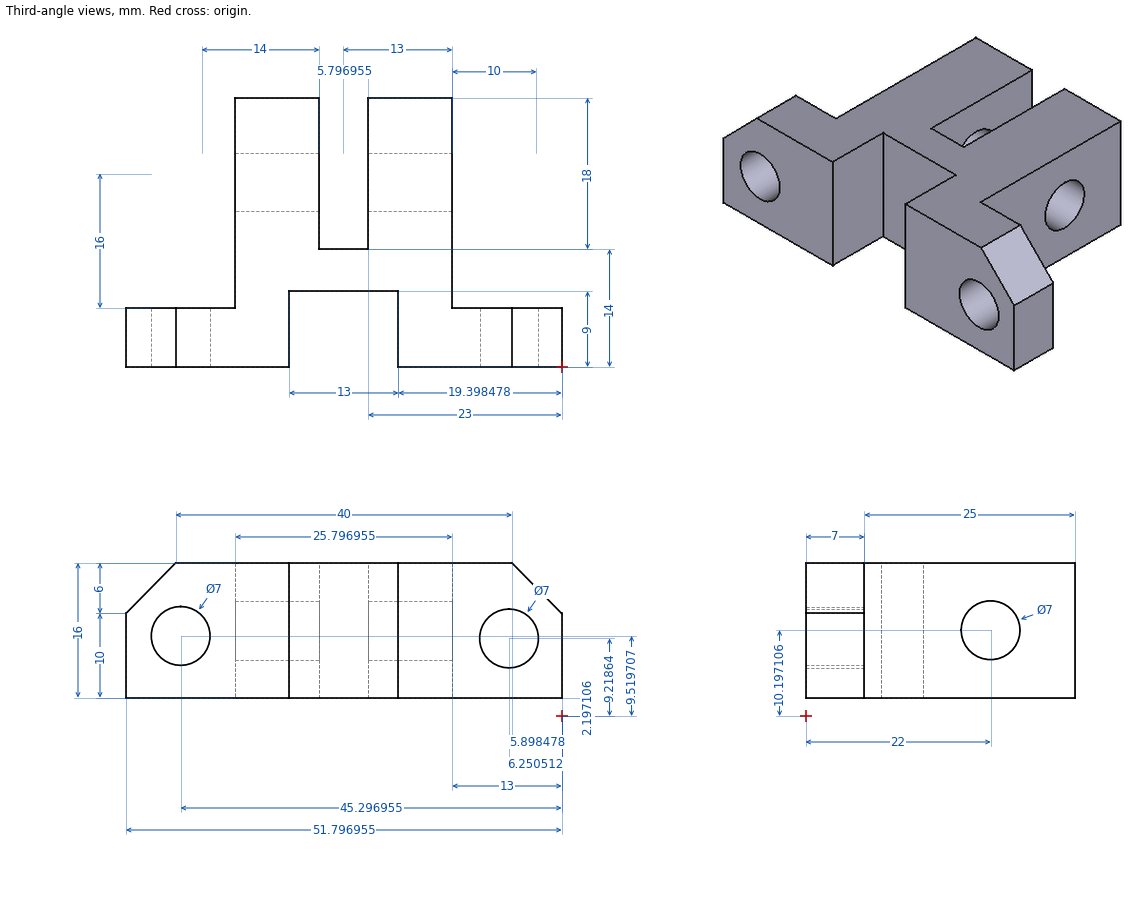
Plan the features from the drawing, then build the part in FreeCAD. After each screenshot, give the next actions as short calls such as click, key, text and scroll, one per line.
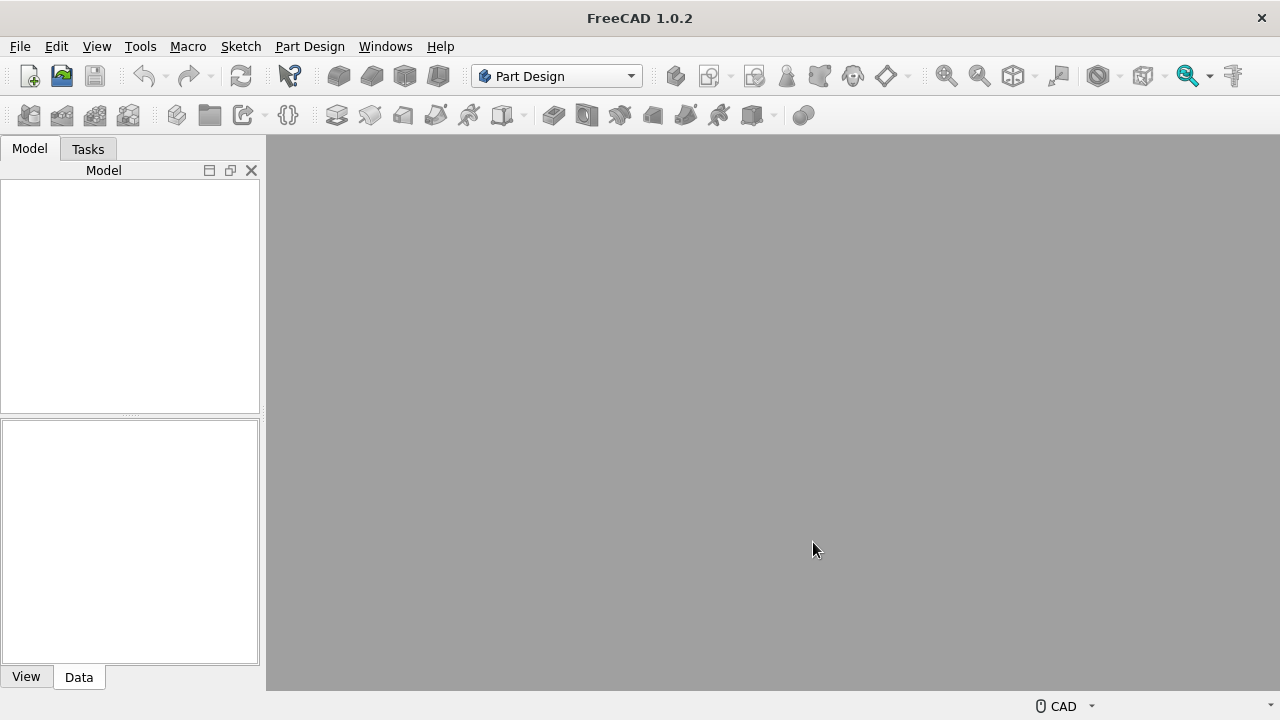
key(ctrl+n)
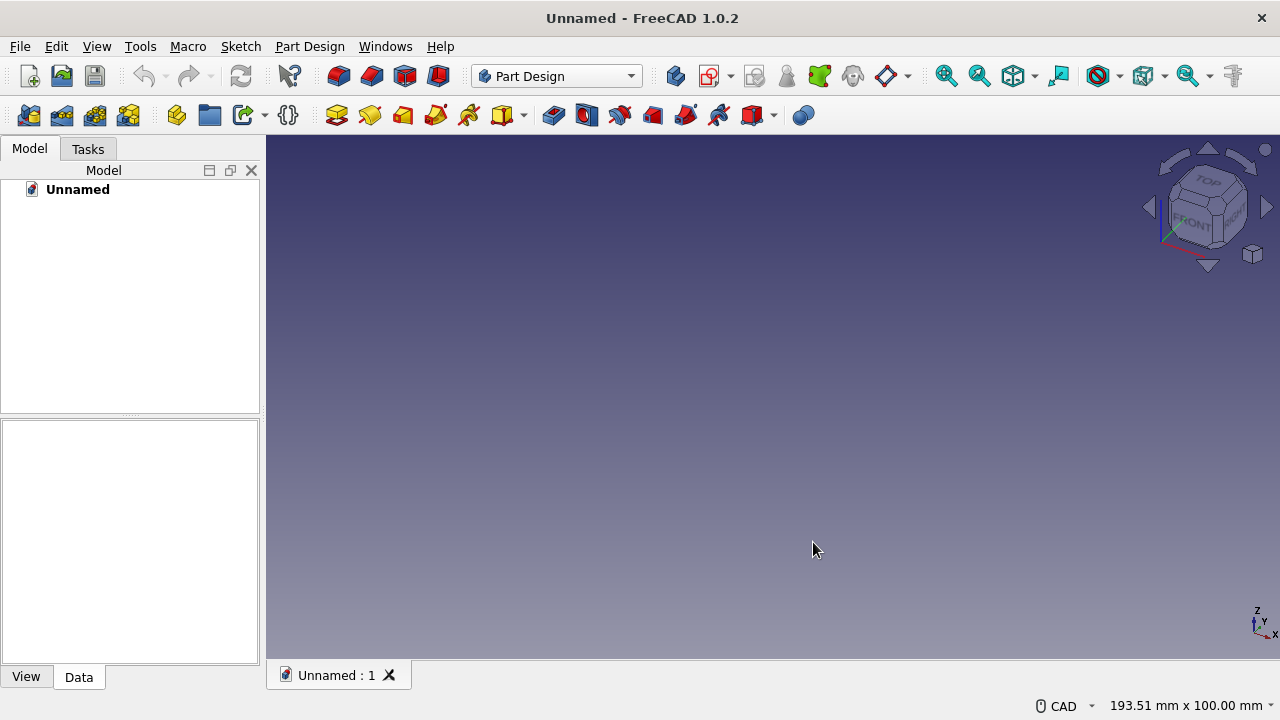
click(708, 76)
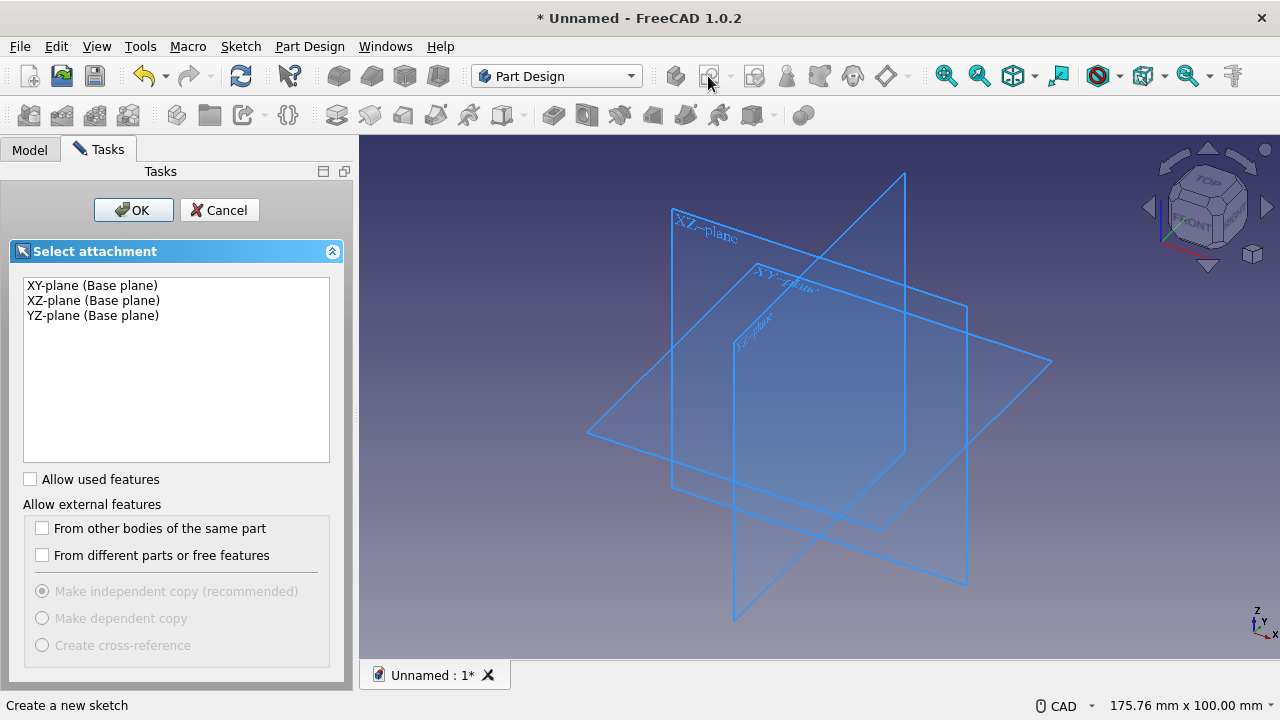
click(84, 300)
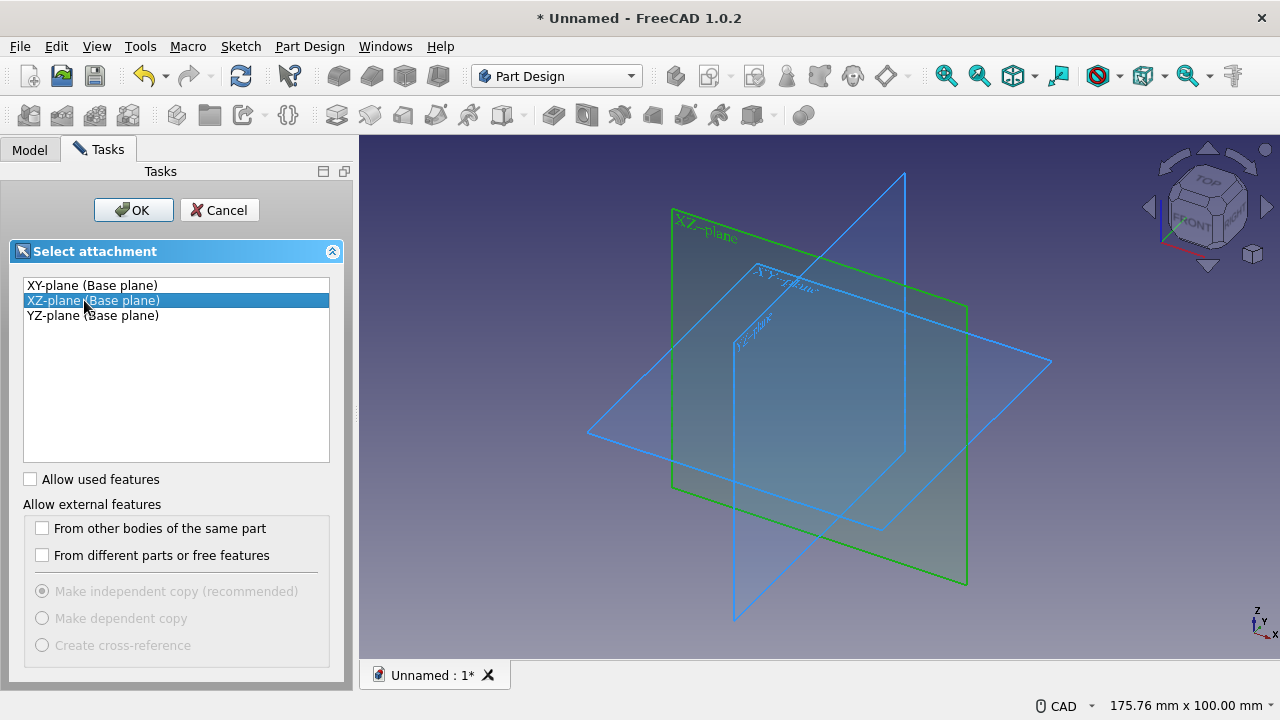
click(134, 210)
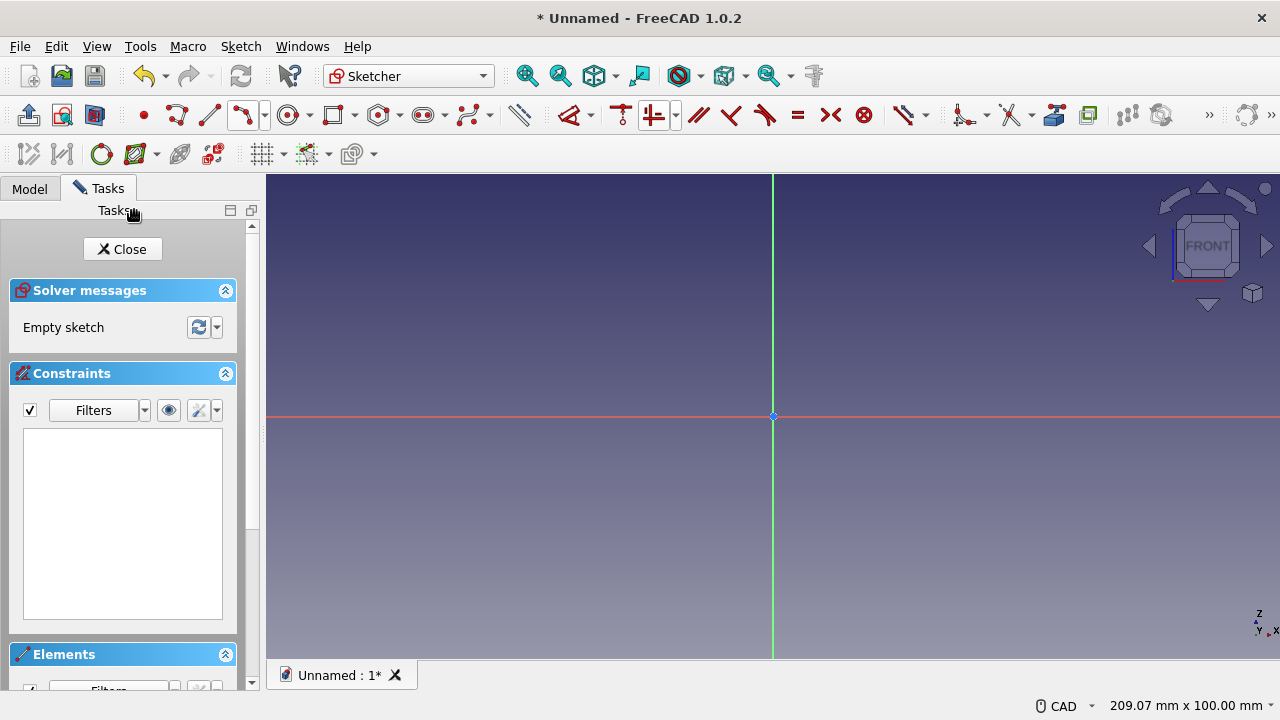
scroll(601, 336, up, 4)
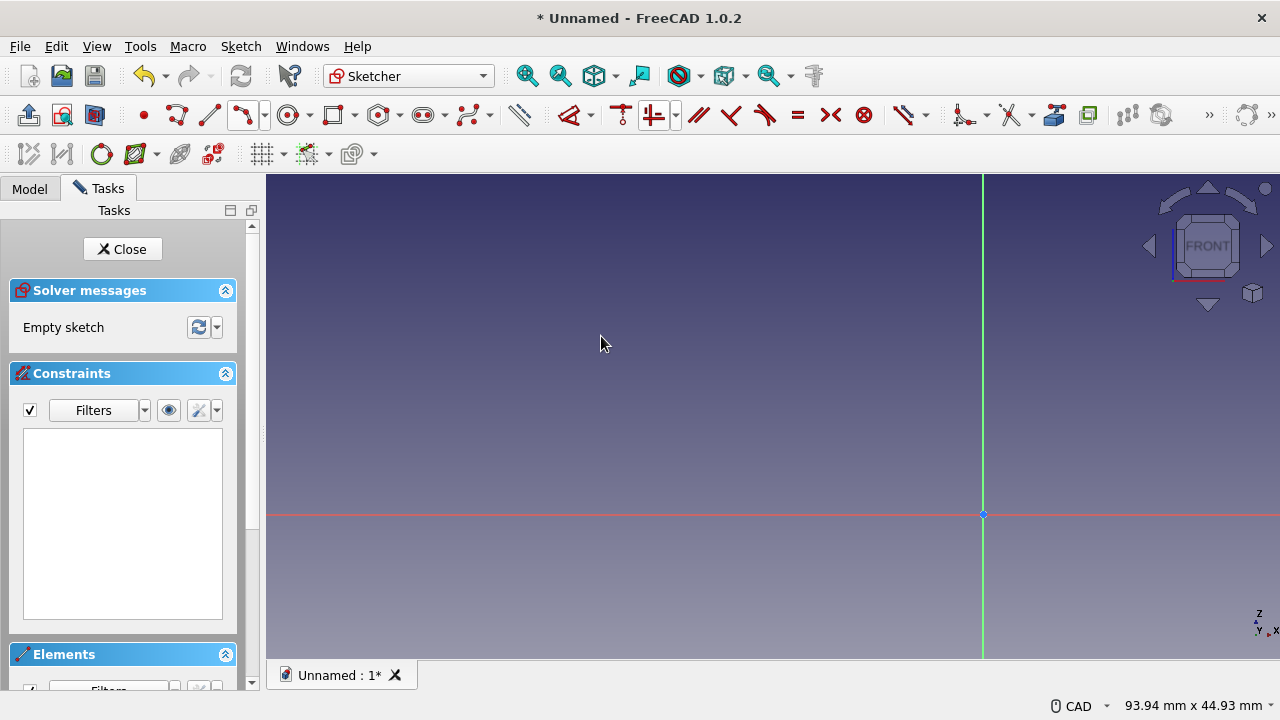
key(g)
key(m)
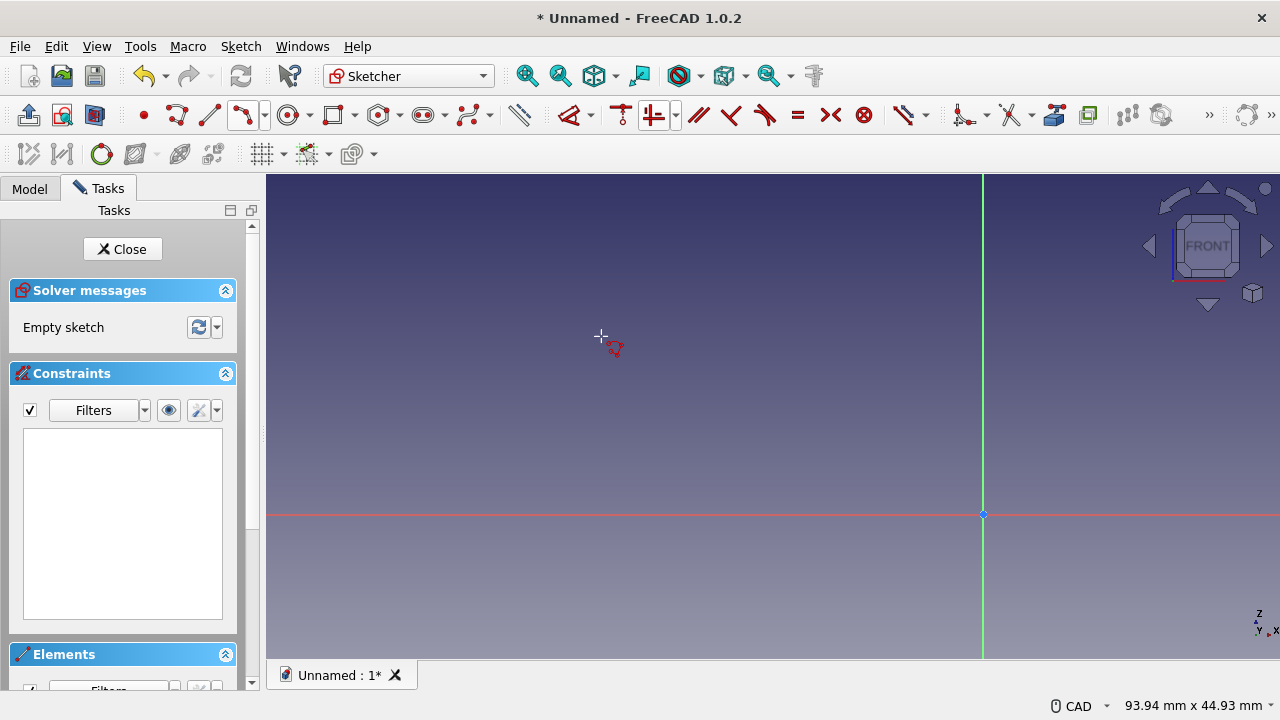
click(983, 491)
click(424, 491)
click(424, 383)
click(488, 318)
click(920, 318)
click(974, 383)
click(983, 492)
key(Escape)
key(Escape)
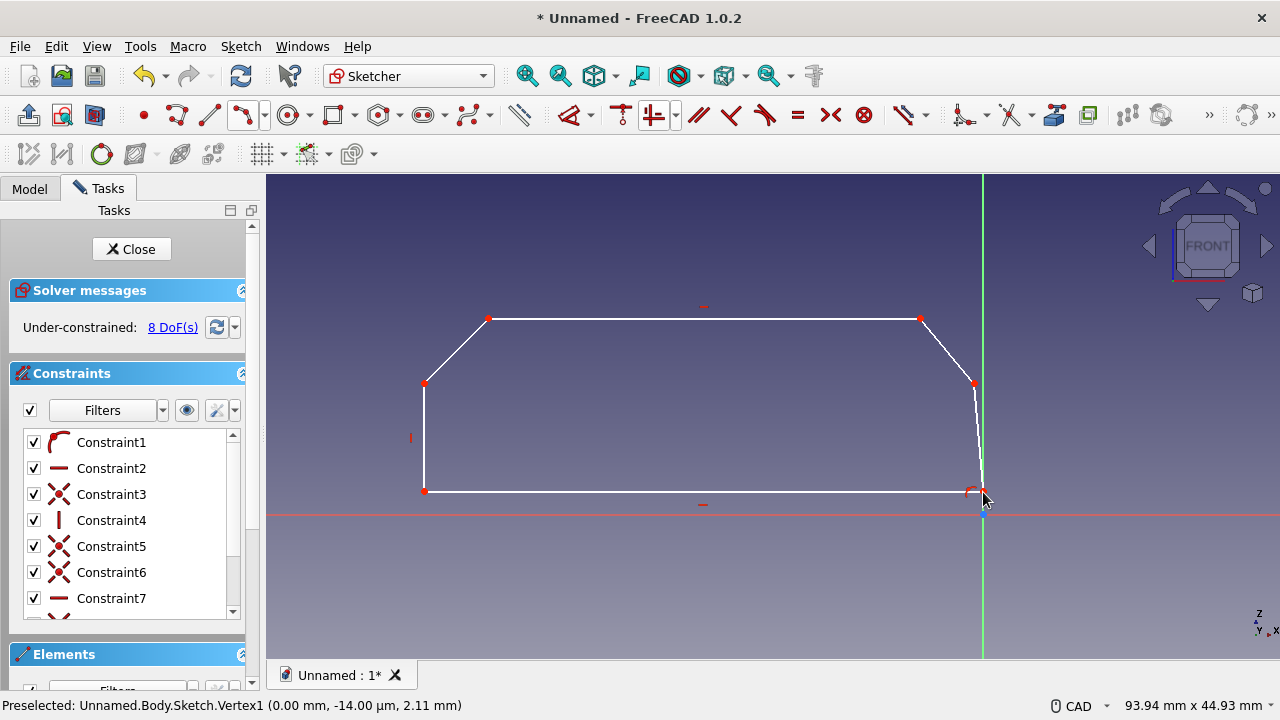
click(981, 460)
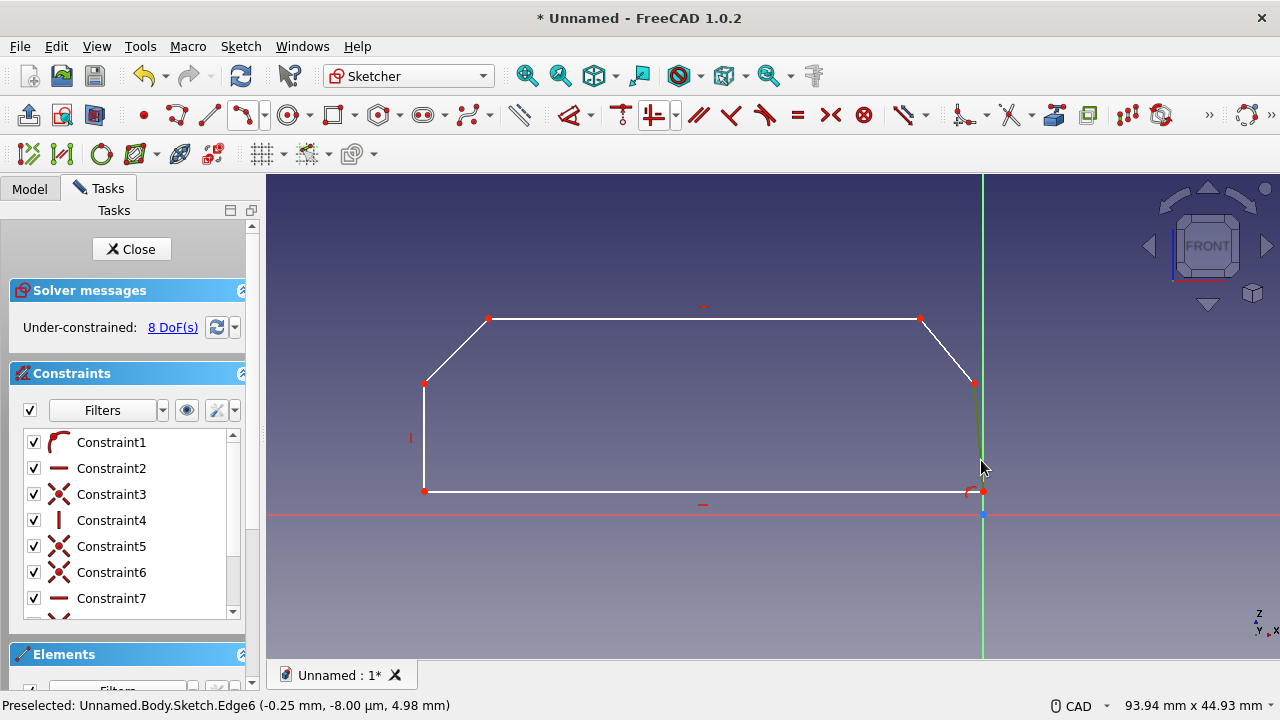
key(v)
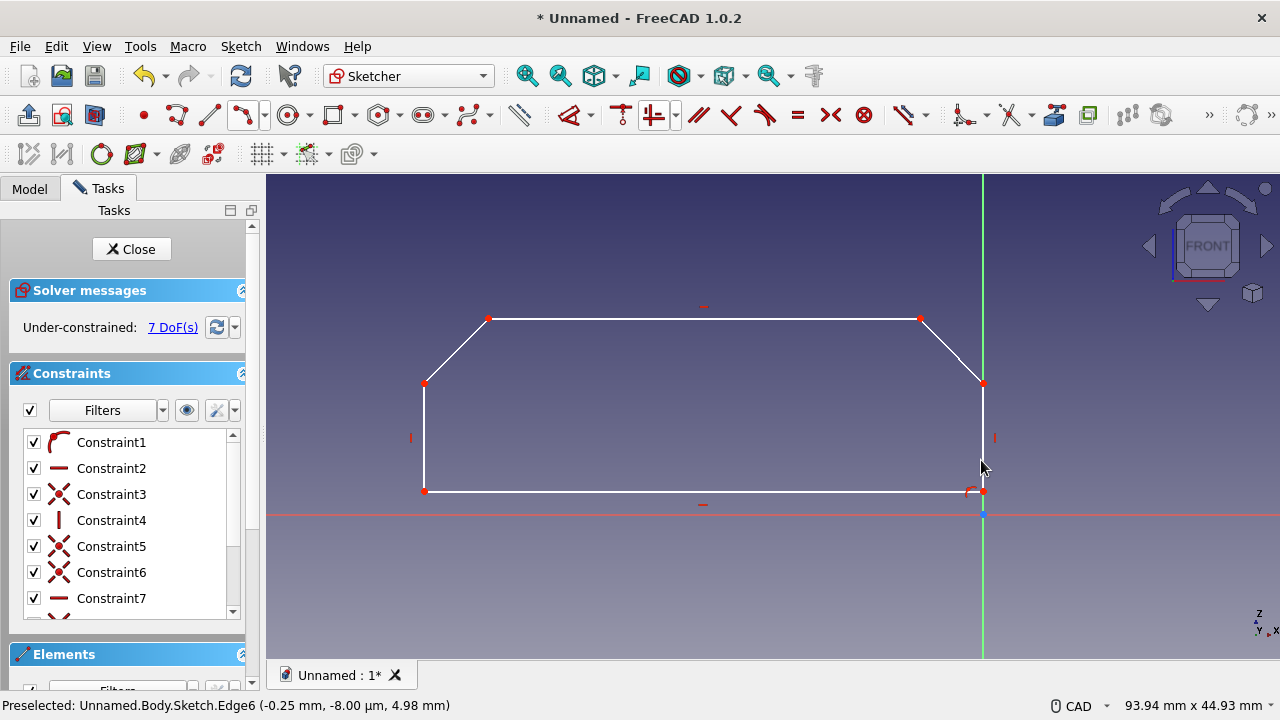
key(d)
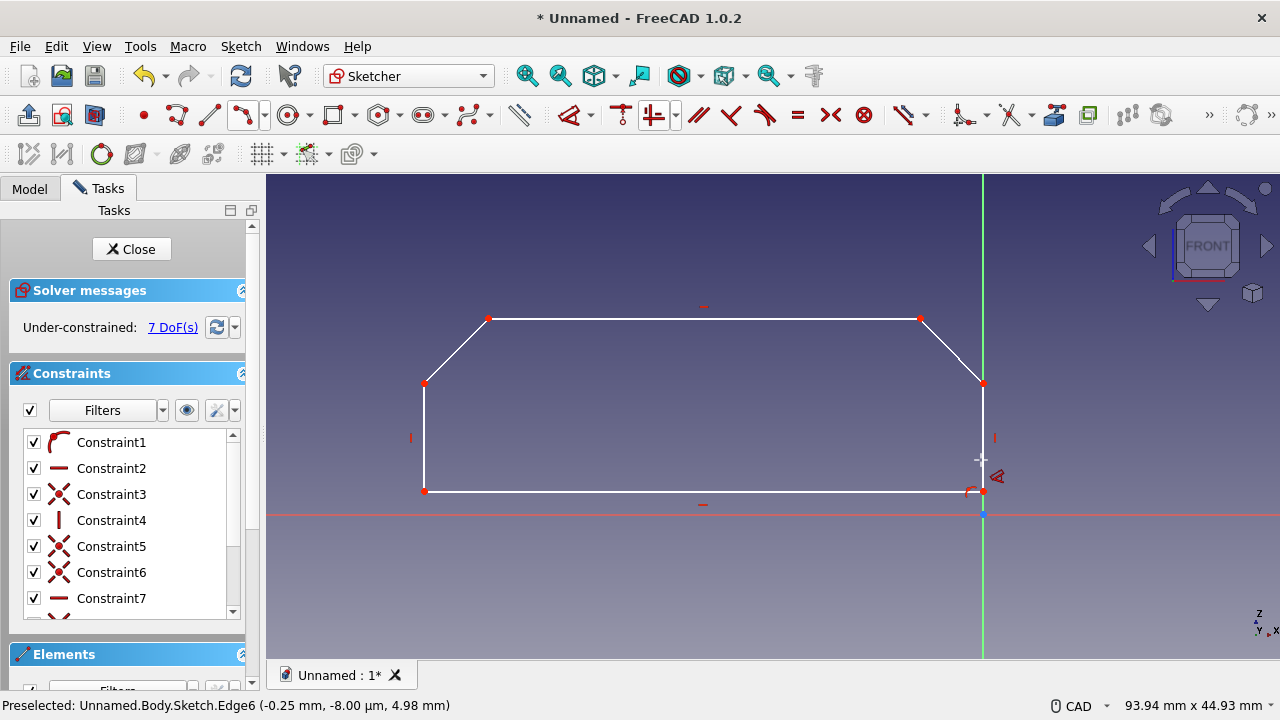
click(424, 460)
click(390, 438)